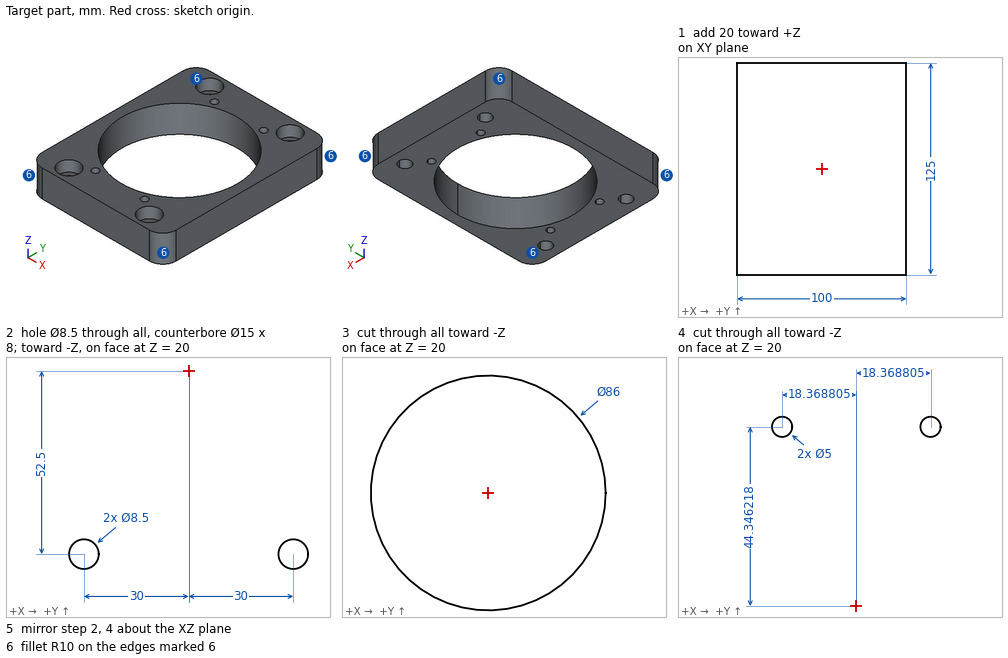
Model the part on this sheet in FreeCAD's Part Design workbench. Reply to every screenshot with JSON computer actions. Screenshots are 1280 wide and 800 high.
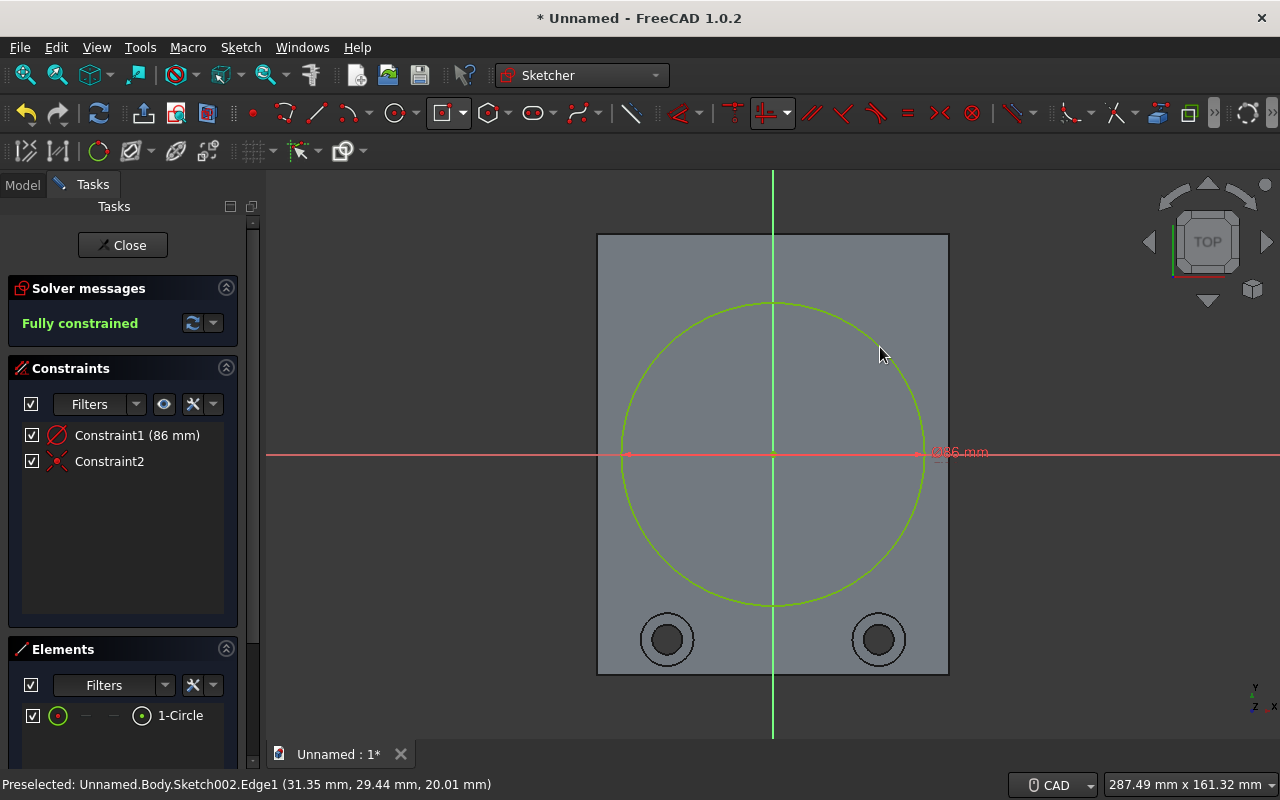
{"action": "left_click", "coordinate": [123, 245]}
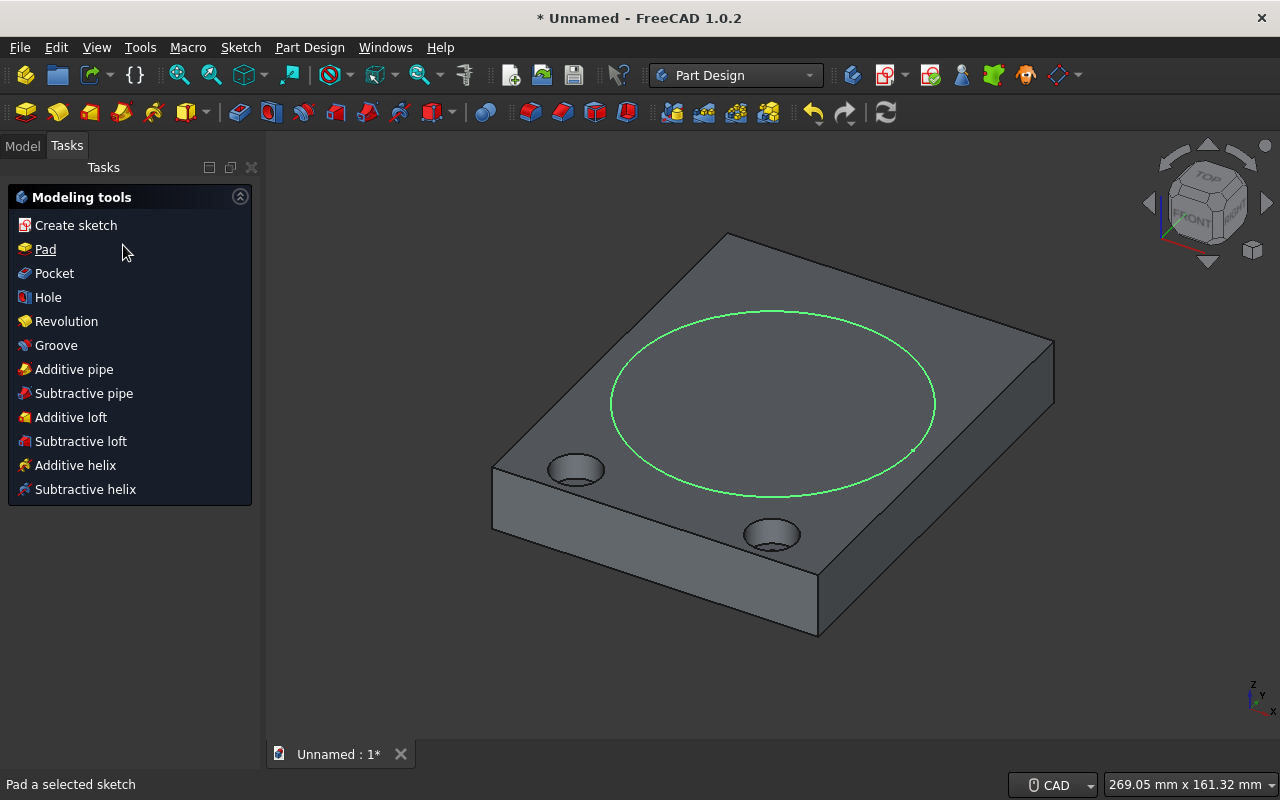
{"action": "left_click", "coordinate": [240, 112]}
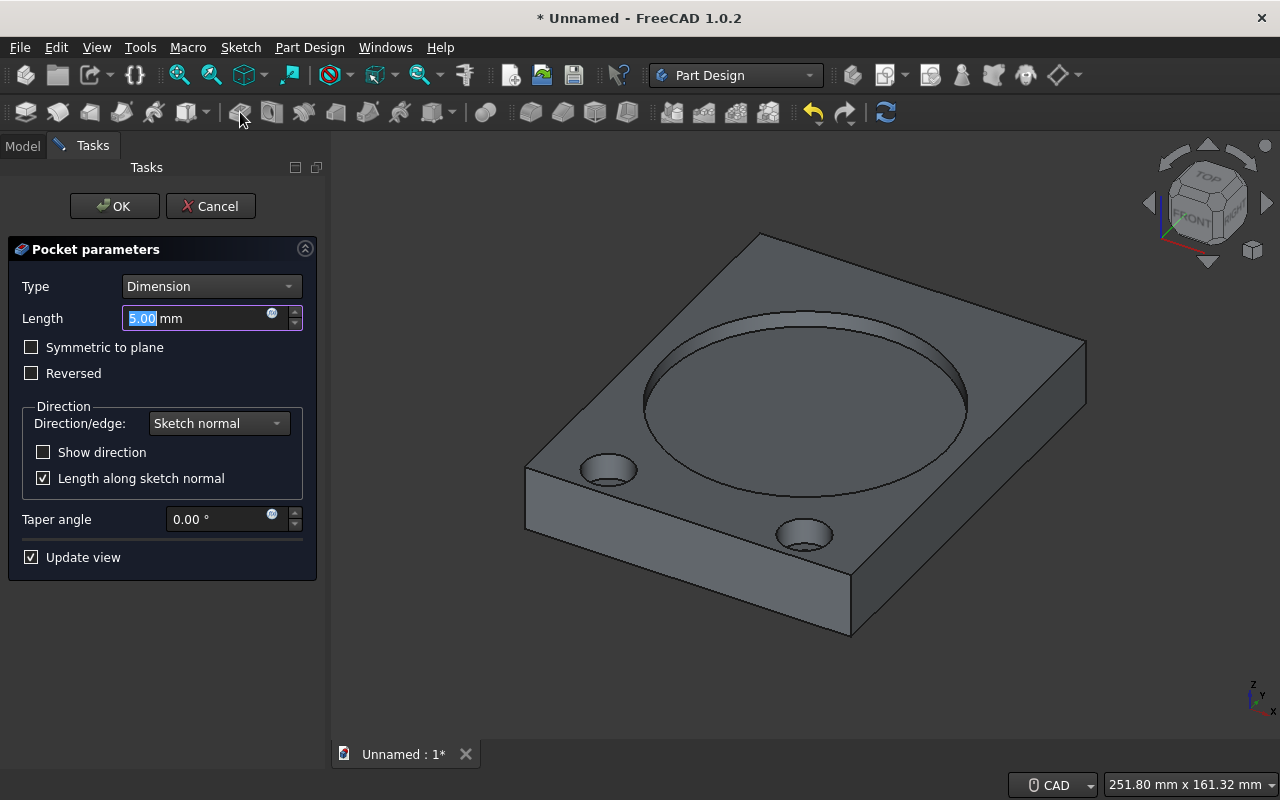
{"action": "left_click", "coordinate": [212, 286]}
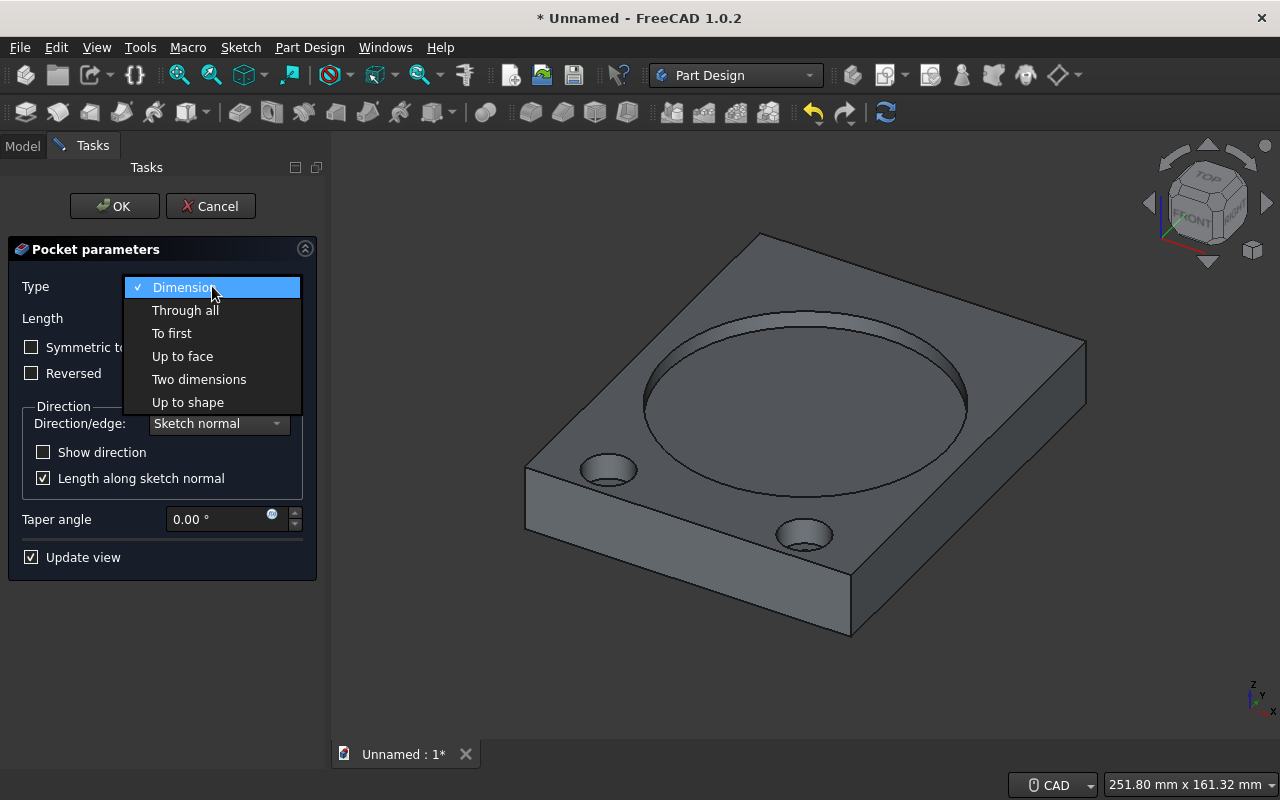
{"action": "left_click", "coordinate": [212, 310]}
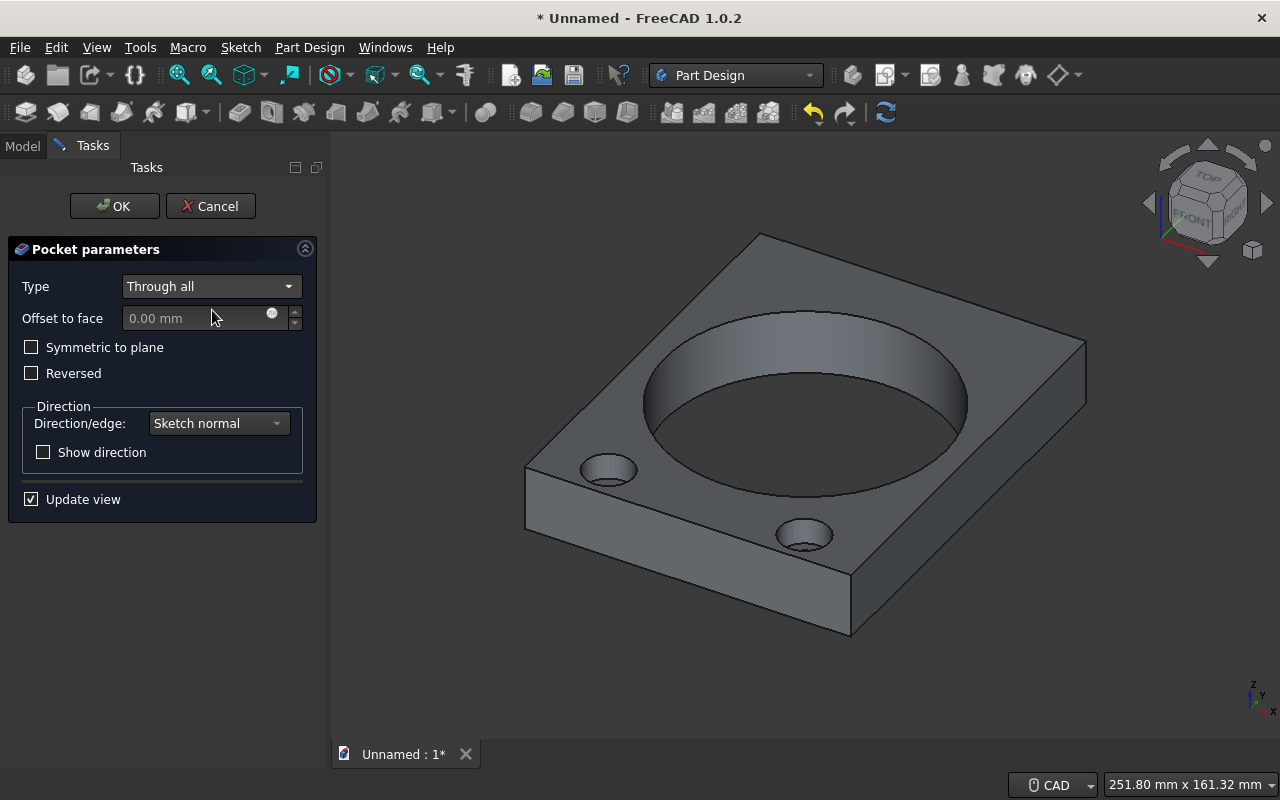
{"action": "left_click", "coordinate": [115, 206]}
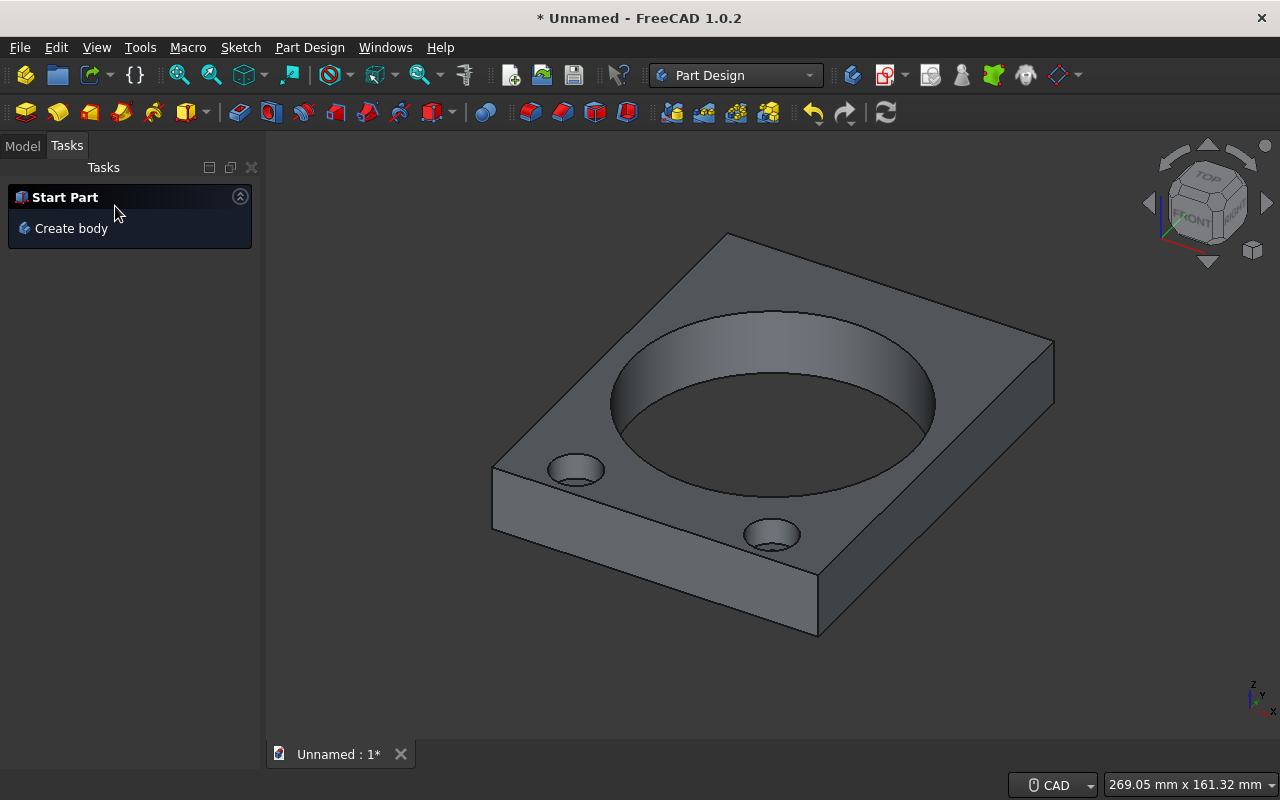
{"action": "left_click", "coordinate": [967, 334]}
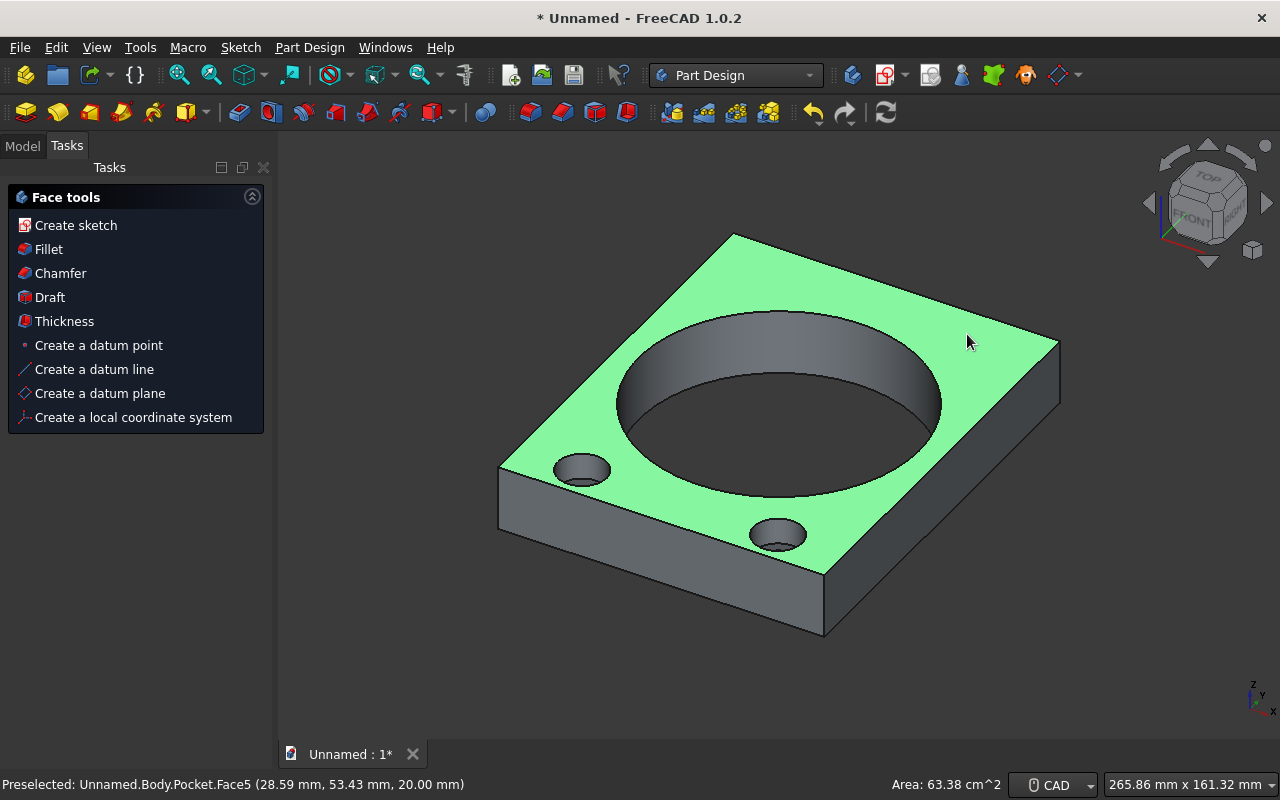
{"action": "left_click", "coordinate": [886, 76]}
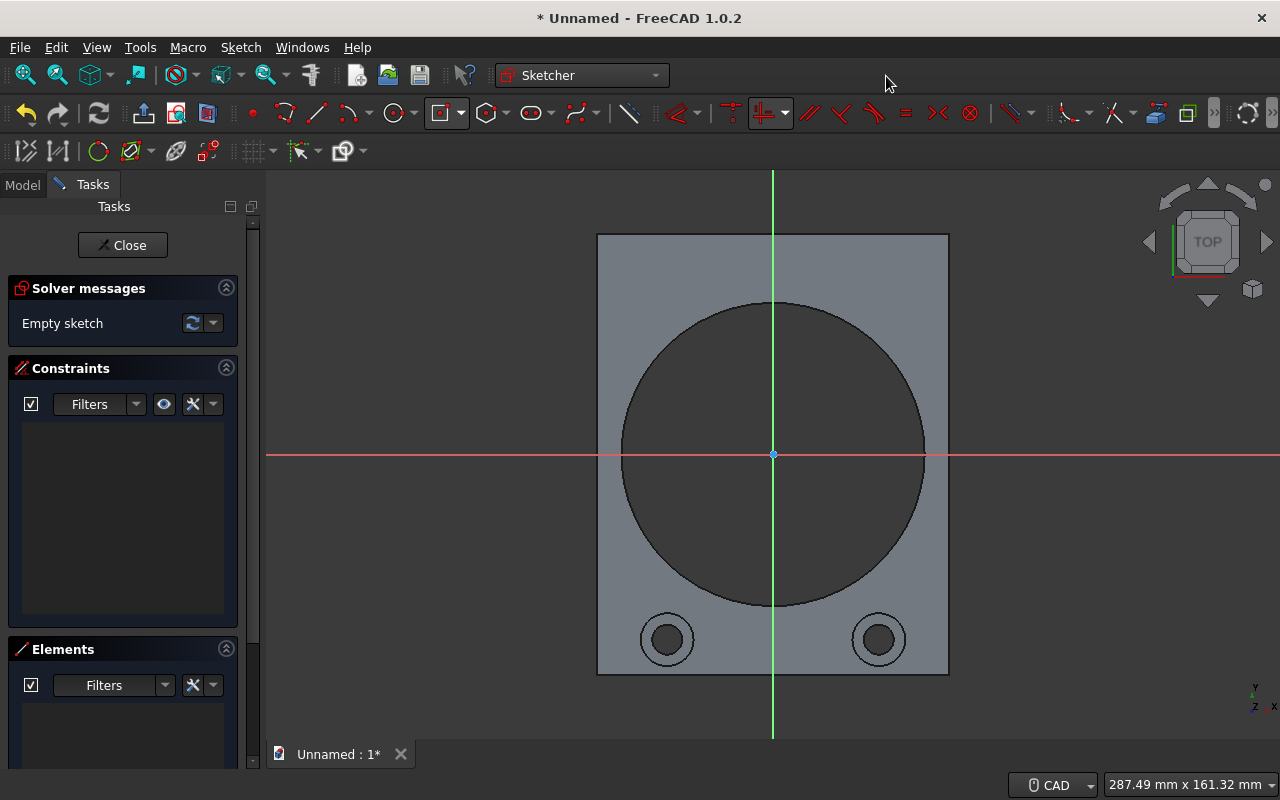
{"action": "scroll", "coordinate": [829, 304], "scroll_direction": "up", "scroll_amount": 4}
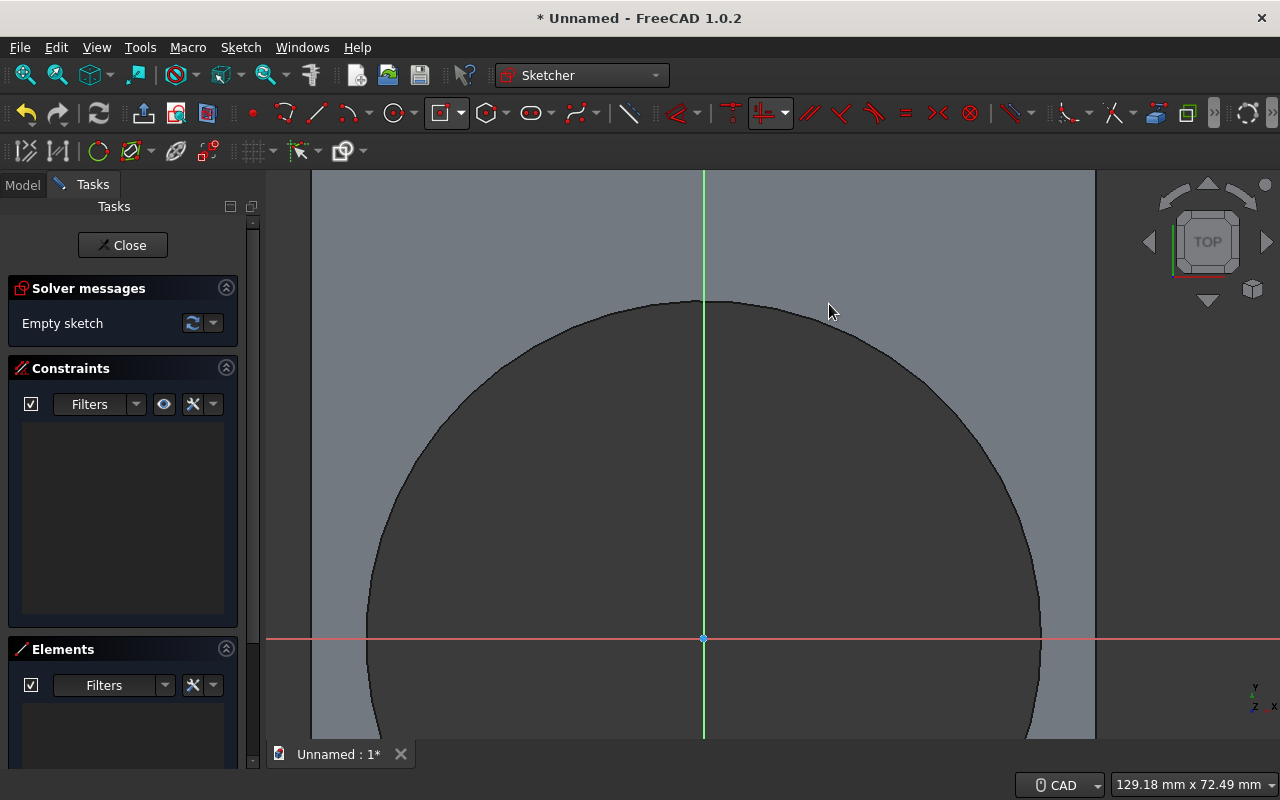
{"action": "left_click", "coordinate": [394, 114]}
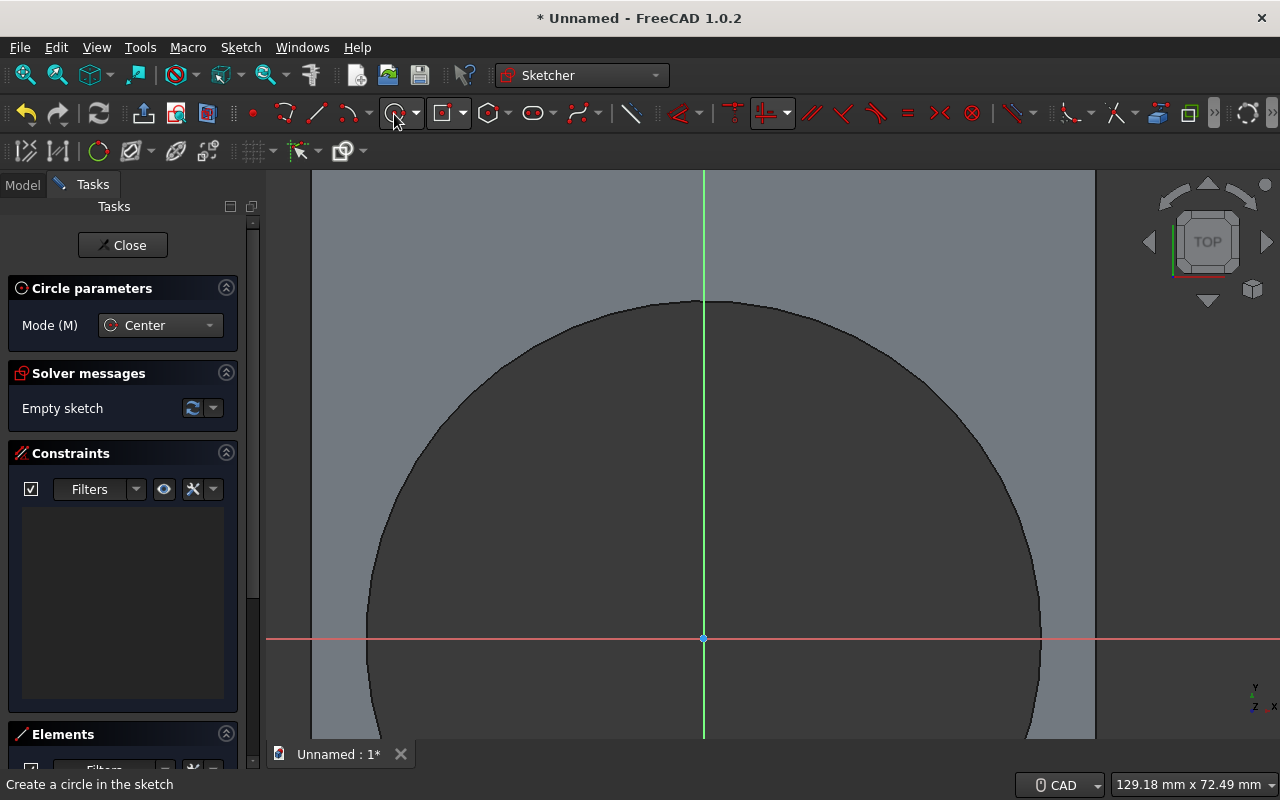
{"action": "left_click", "coordinate": [559, 291]}
{"action": "mouse_move", "coordinate": [573, 277]}